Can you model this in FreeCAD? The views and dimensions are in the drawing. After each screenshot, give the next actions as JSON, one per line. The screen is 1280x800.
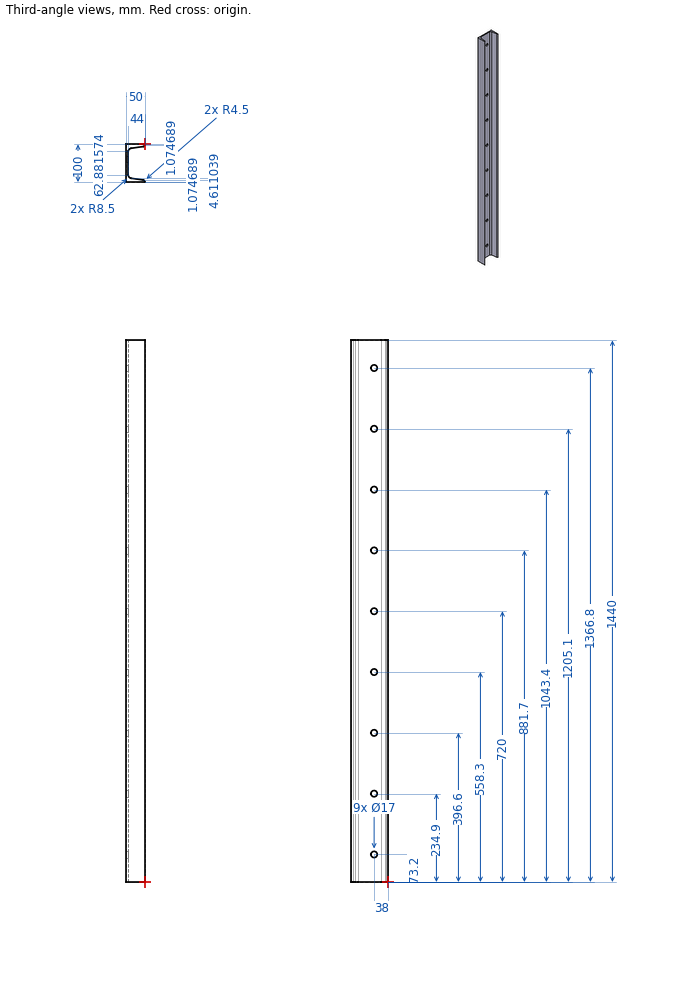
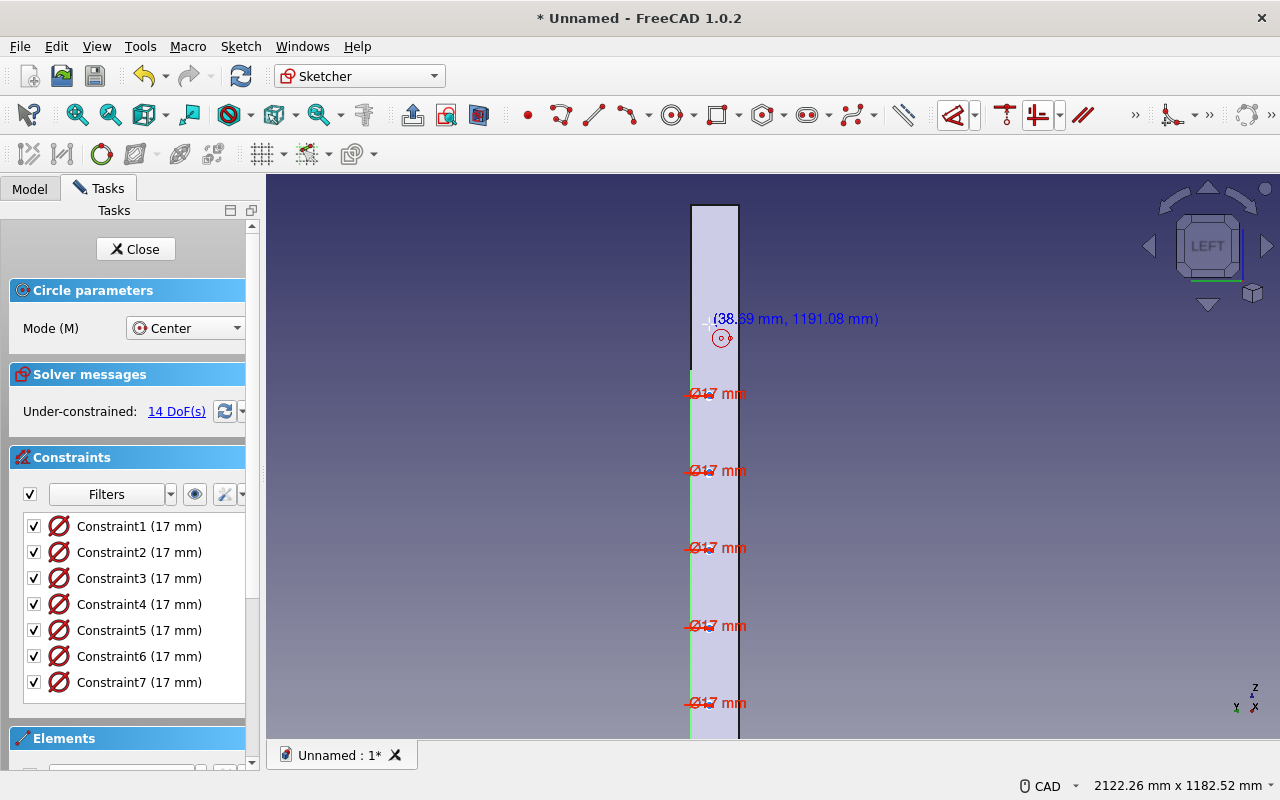
{"action": "scroll", "coordinate": [709, 321], "scroll_direction": "up", "scroll_amount": 3}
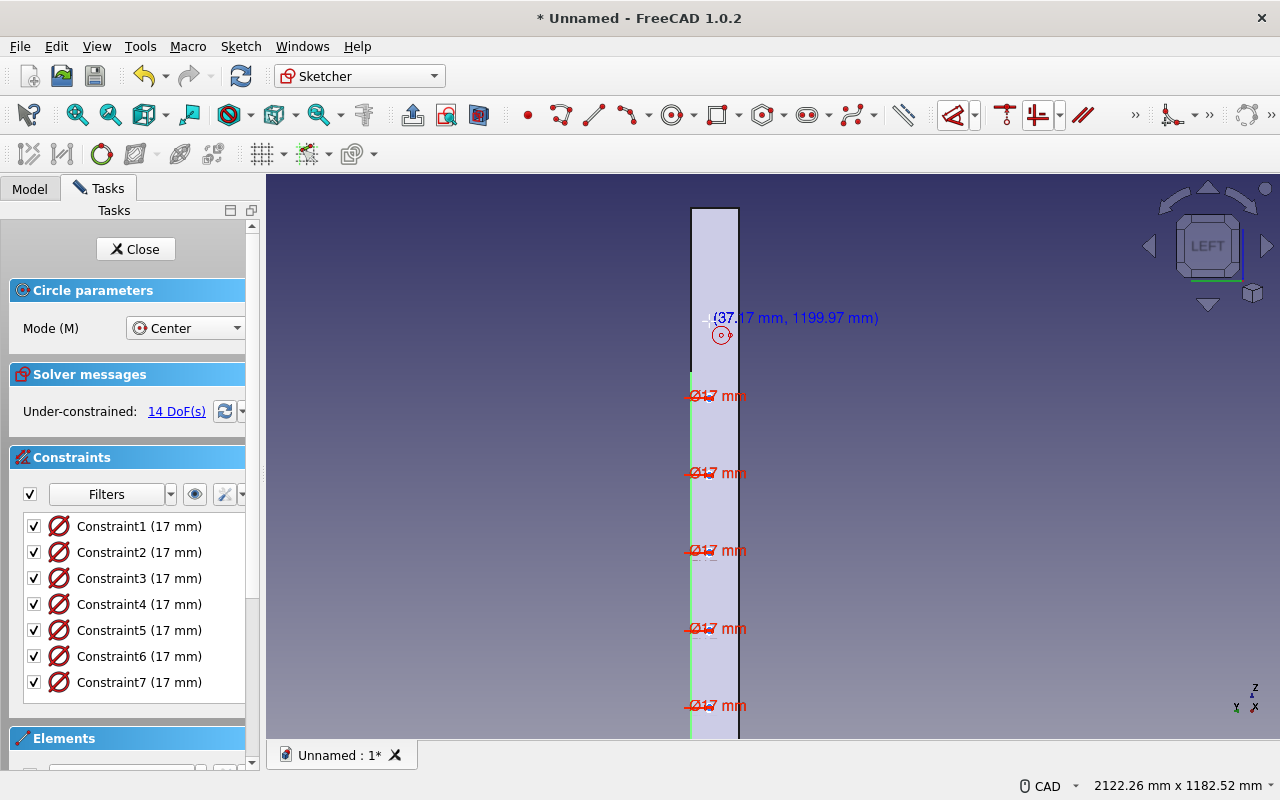
{"action": "left_click", "coordinate": [709, 320]}
{"action": "mouse_move", "coordinate": [712, 317]}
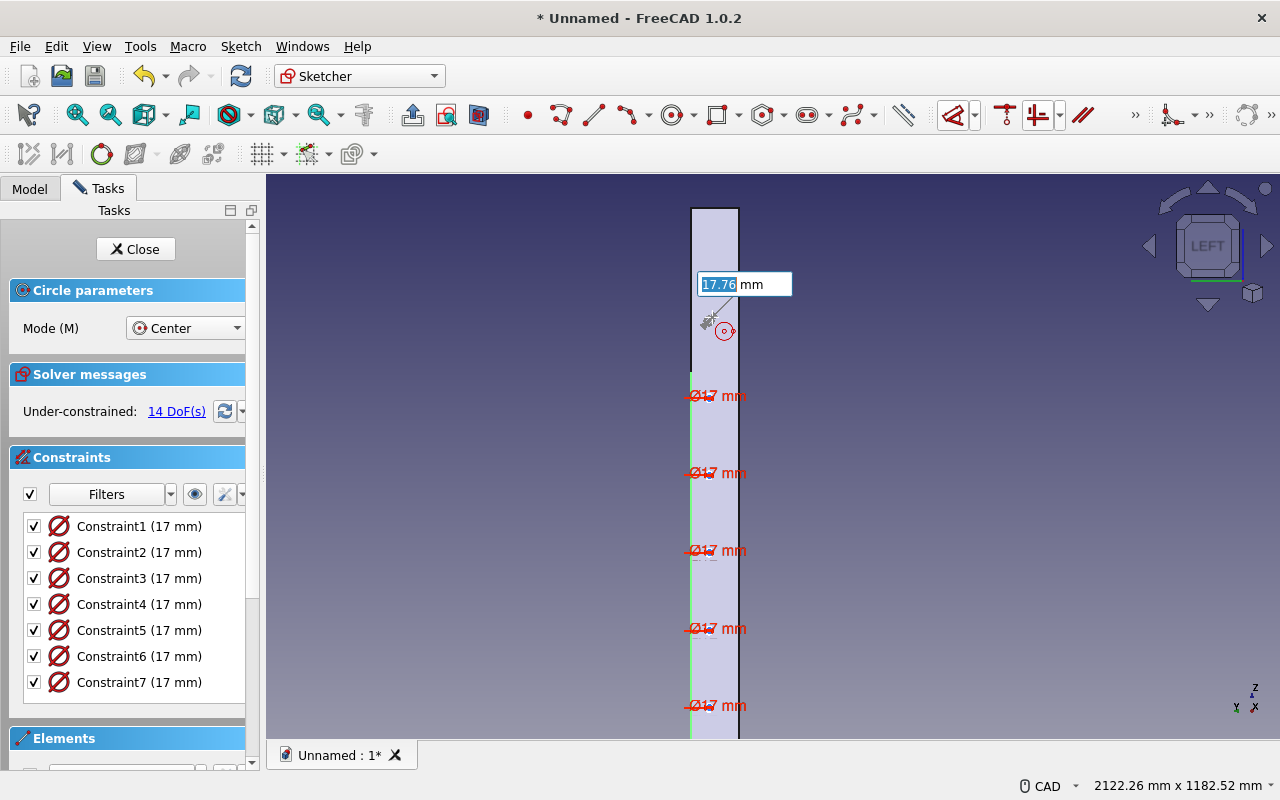
{"action": "type", "text": "17"}
{"action": "key", "text": "Return"}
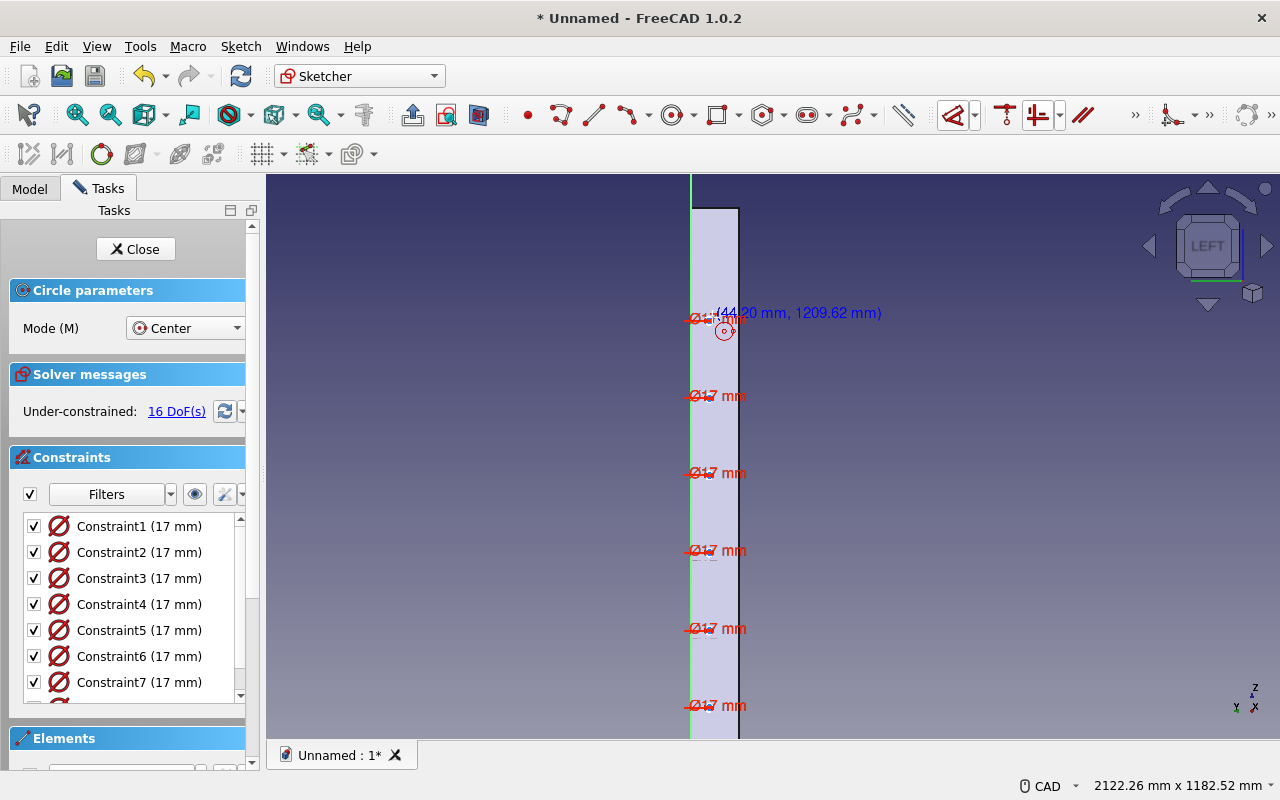
{"action": "scroll", "coordinate": [709, 243], "scroll_direction": "up", "scroll_amount": 9}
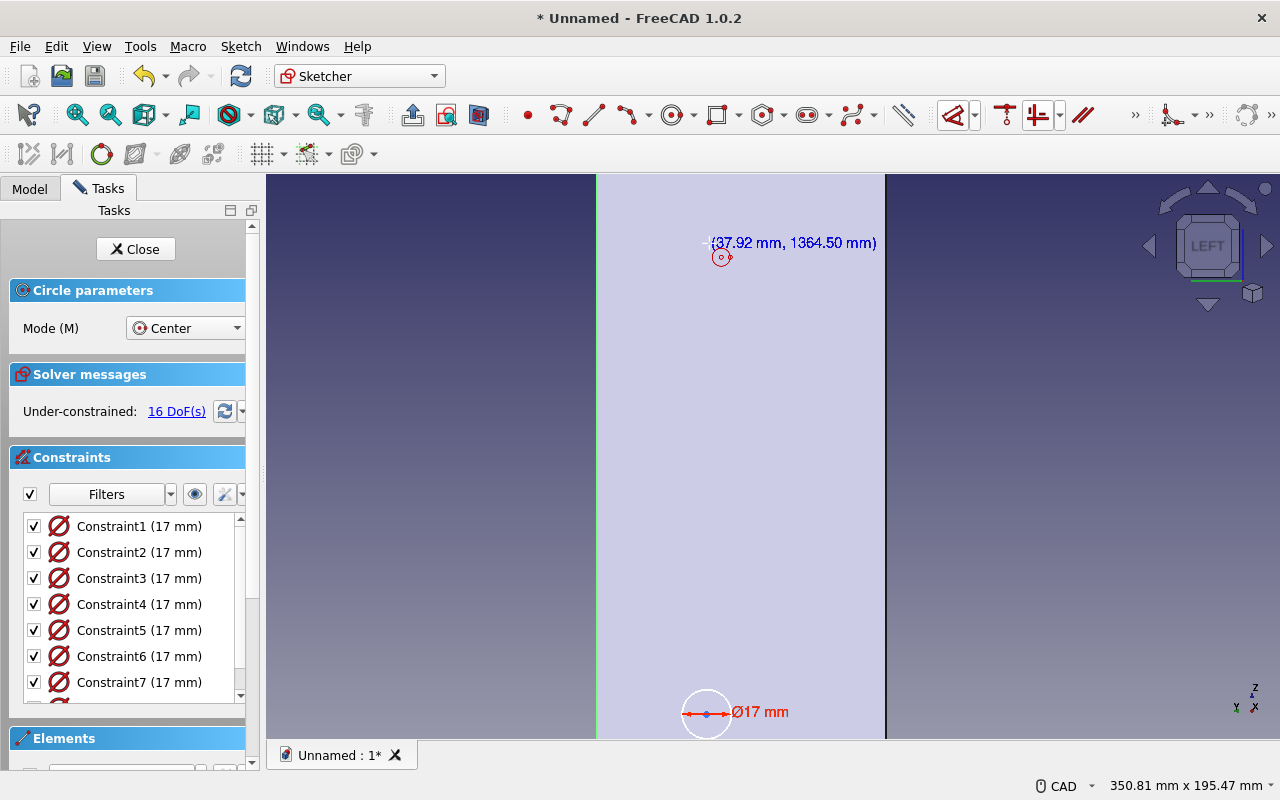
{"action": "scroll", "coordinate": [709, 282], "scroll_direction": "down", "scroll_amount": 12}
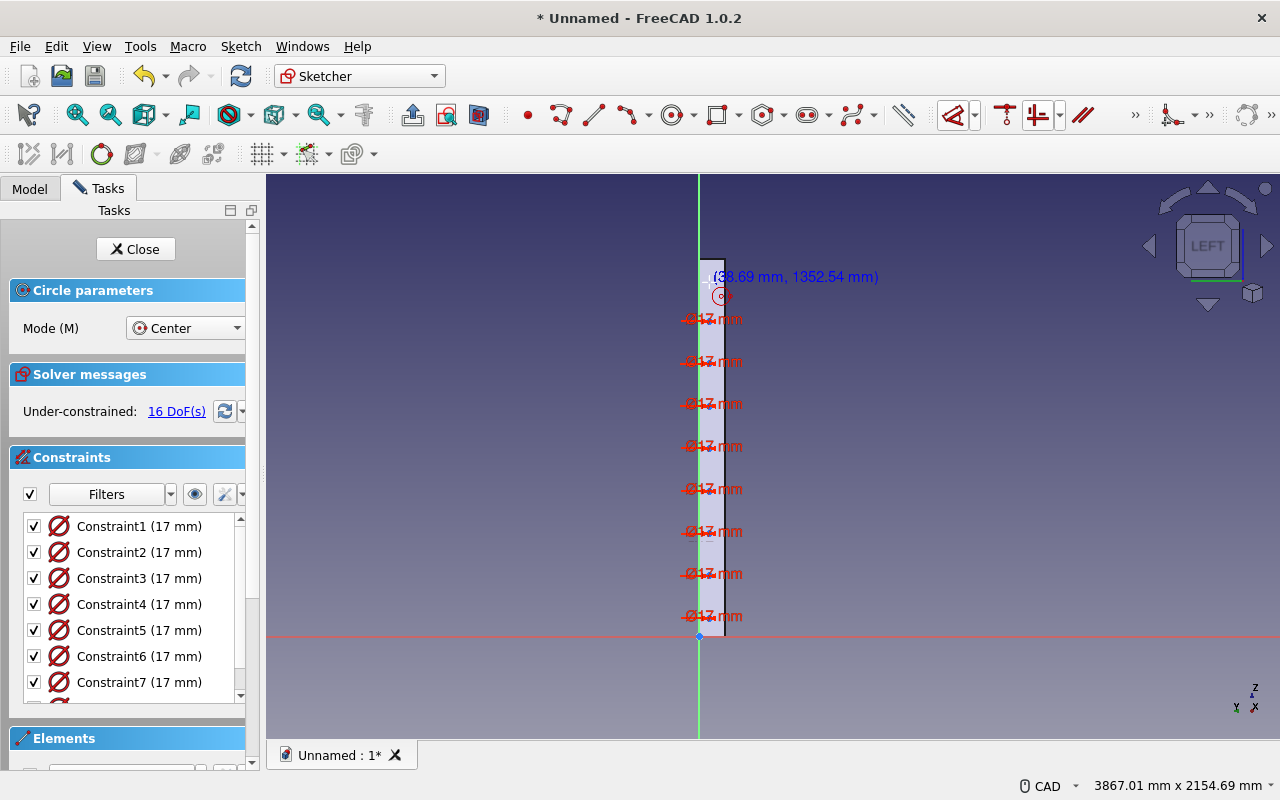
{"action": "scroll", "coordinate": [709, 279], "scroll_direction": "up", "scroll_amount": 3}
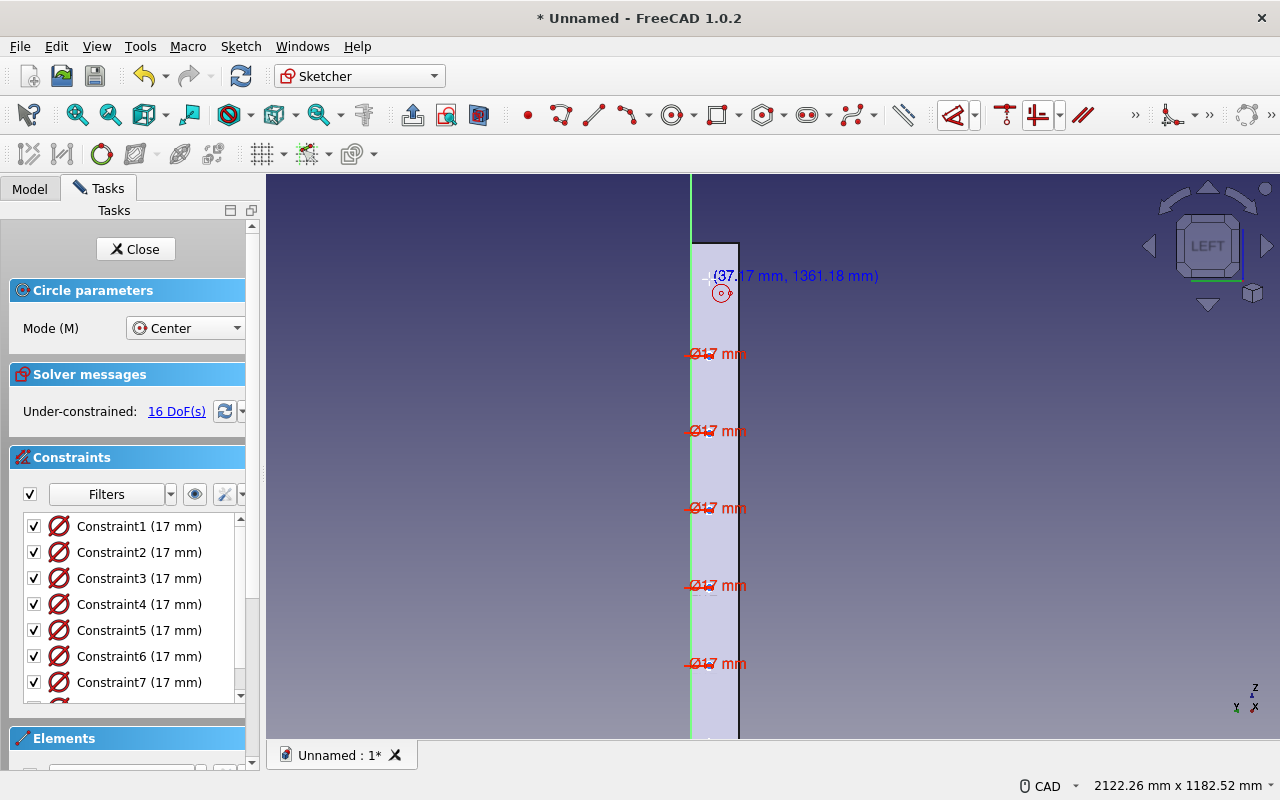
{"action": "left_click", "coordinate": [709, 278]}
{"action": "mouse_move", "coordinate": [712, 275]}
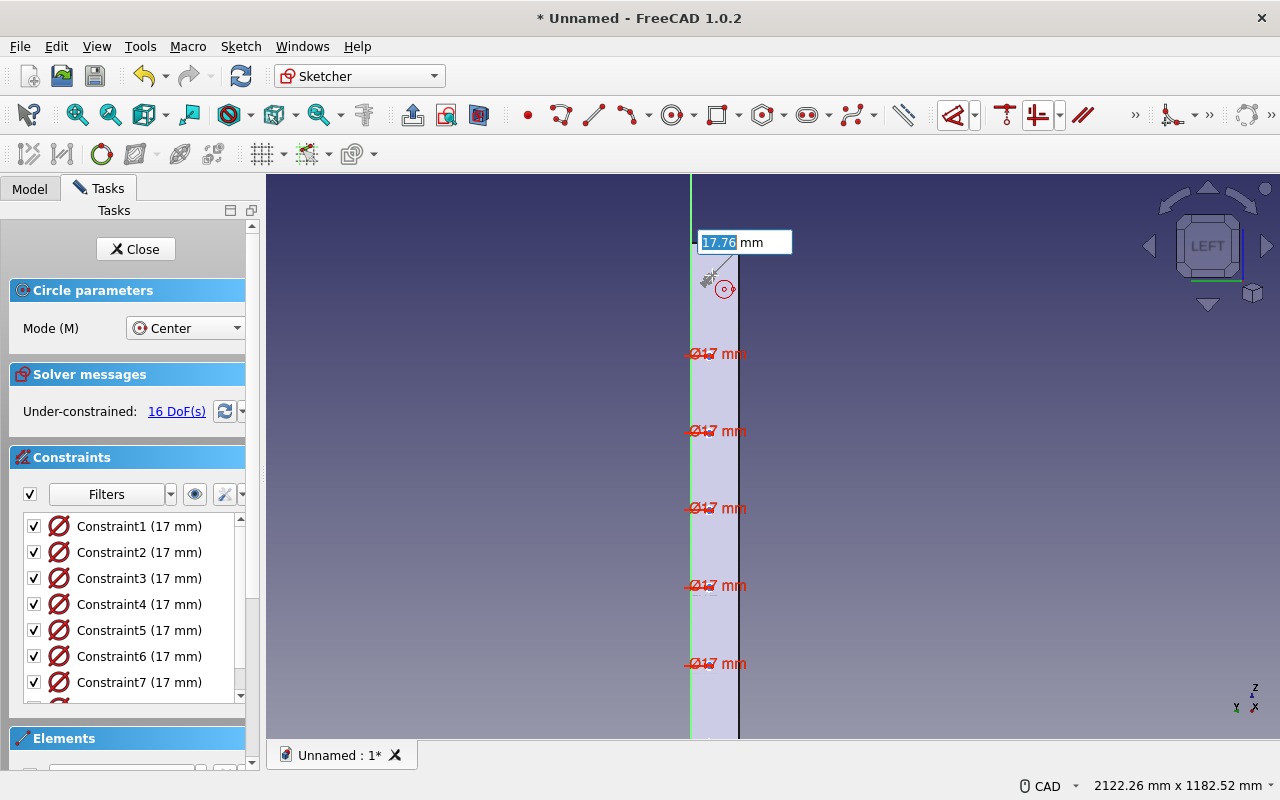
{"action": "type", "text": "17"}
{"action": "key", "text": "Return"}
{"action": "key", "text": "Escape"}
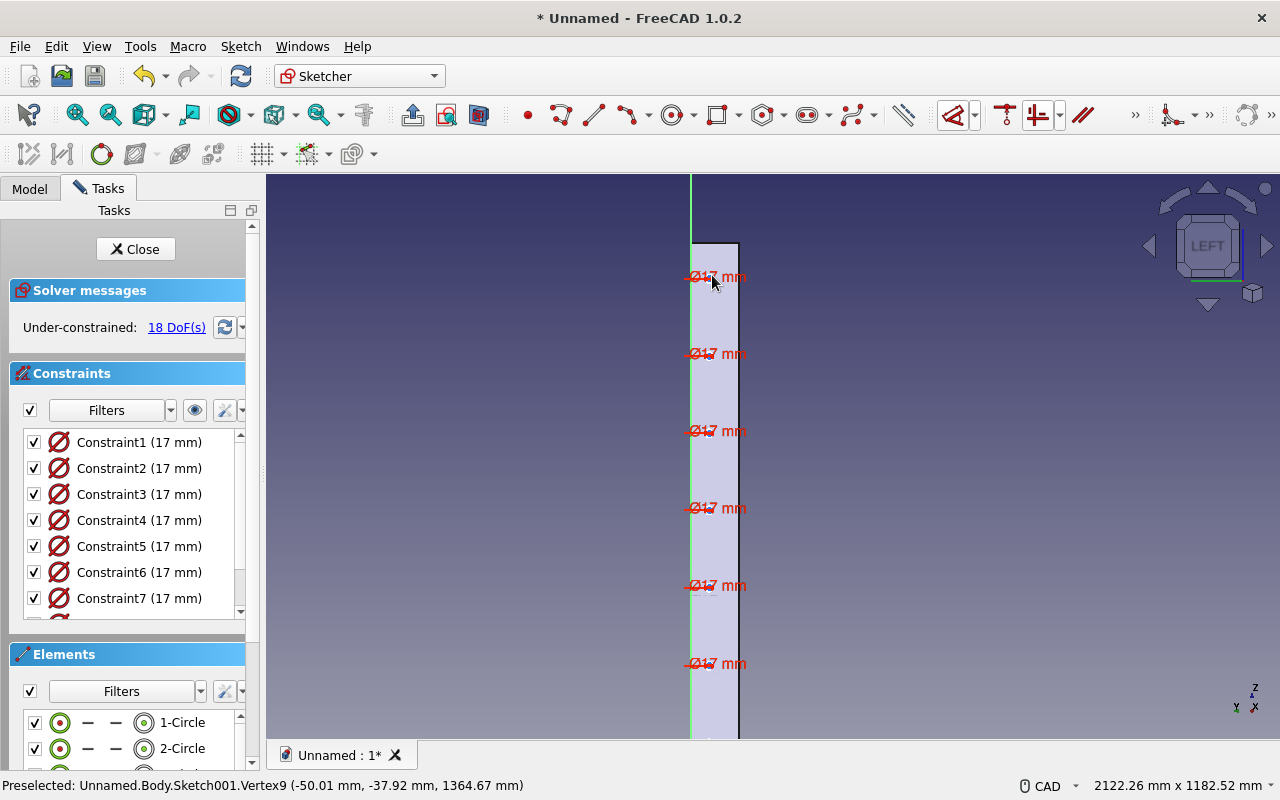
{"action": "scroll", "coordinate": [708, 279], "scroll_direction": "down", "scroll_amount": 3}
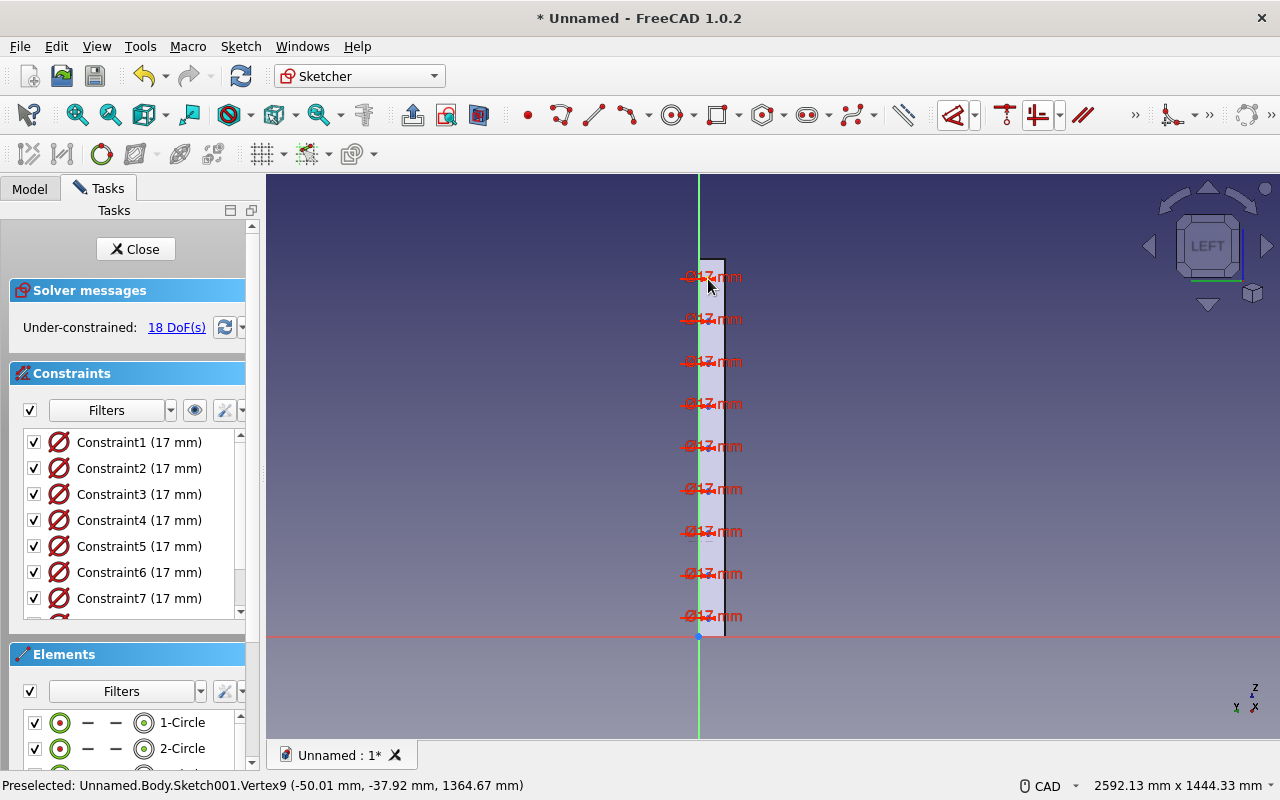
{"action": "scroll", "coordinate": [709, 618], "scroll_direction": "up", "scroll_amount": 7}